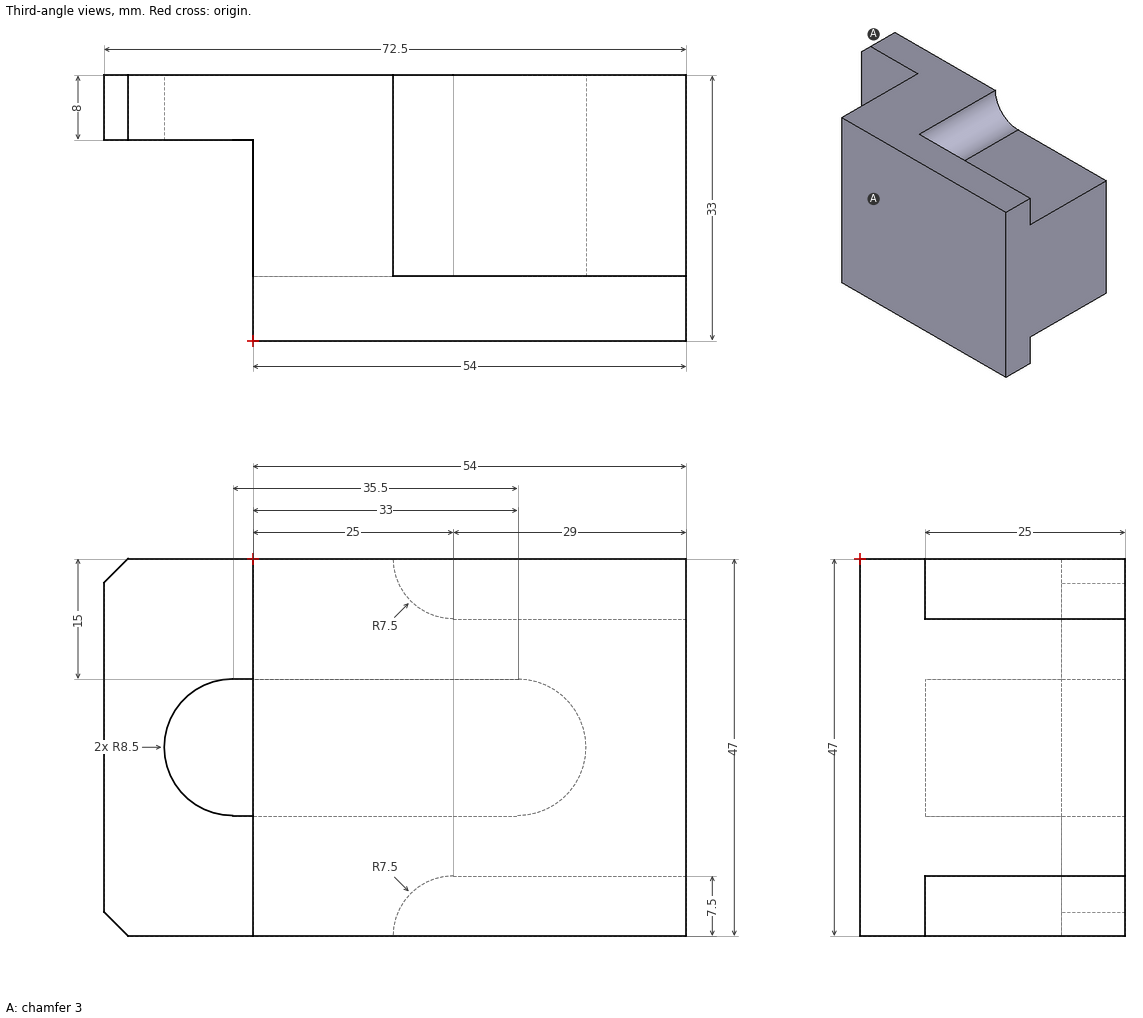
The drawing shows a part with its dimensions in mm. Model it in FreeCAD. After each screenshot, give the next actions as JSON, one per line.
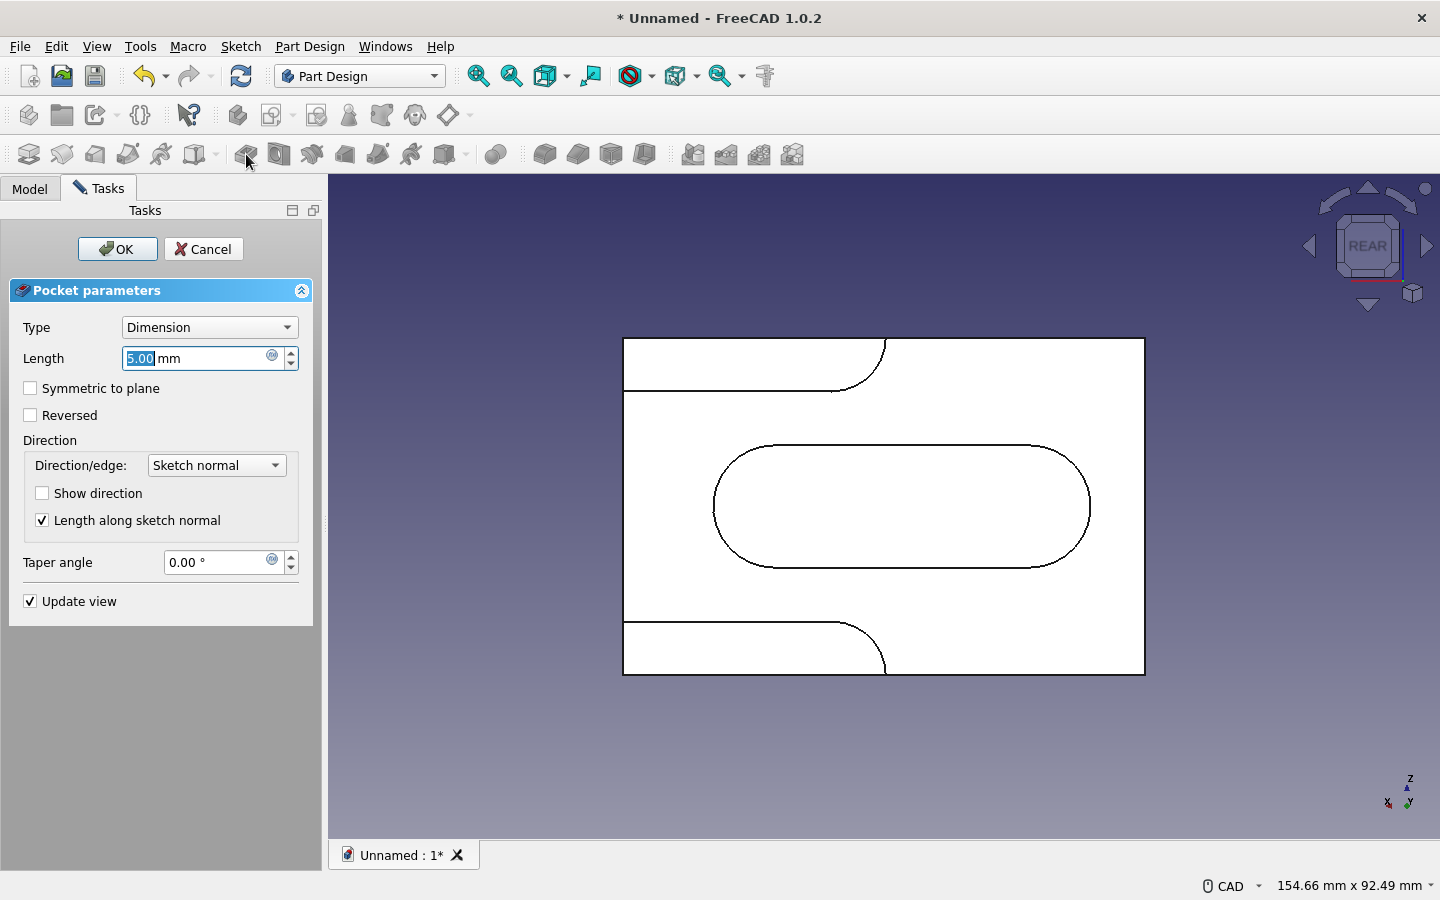
{"action": "type", "text": "25"}
{"action": "key", "text": "Tab"}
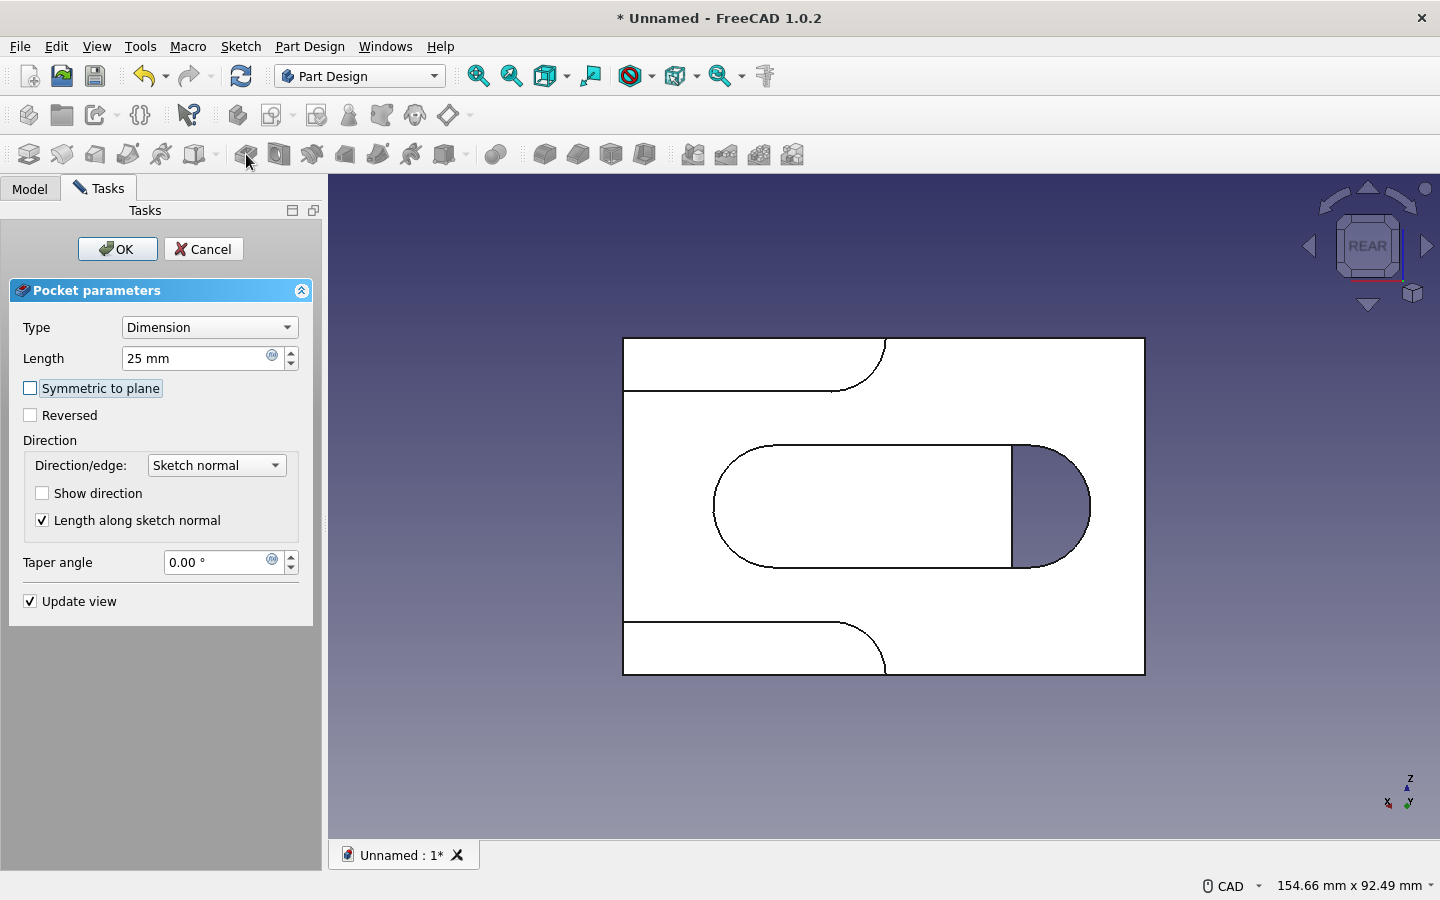
{"action": "left_click", "coordinate": [118, 249]}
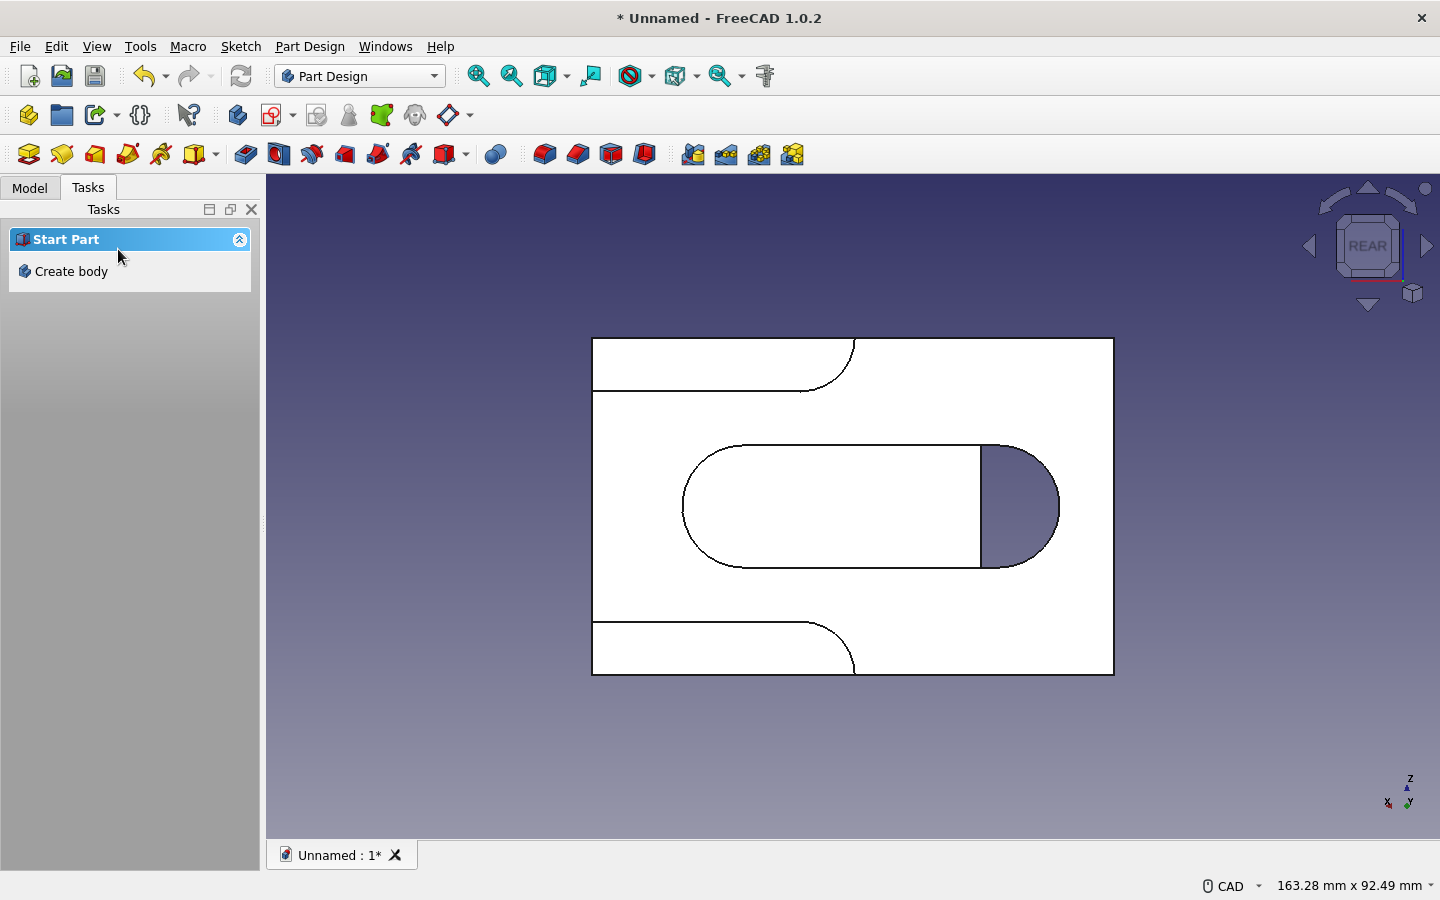
{"action": "key", "text": "0"}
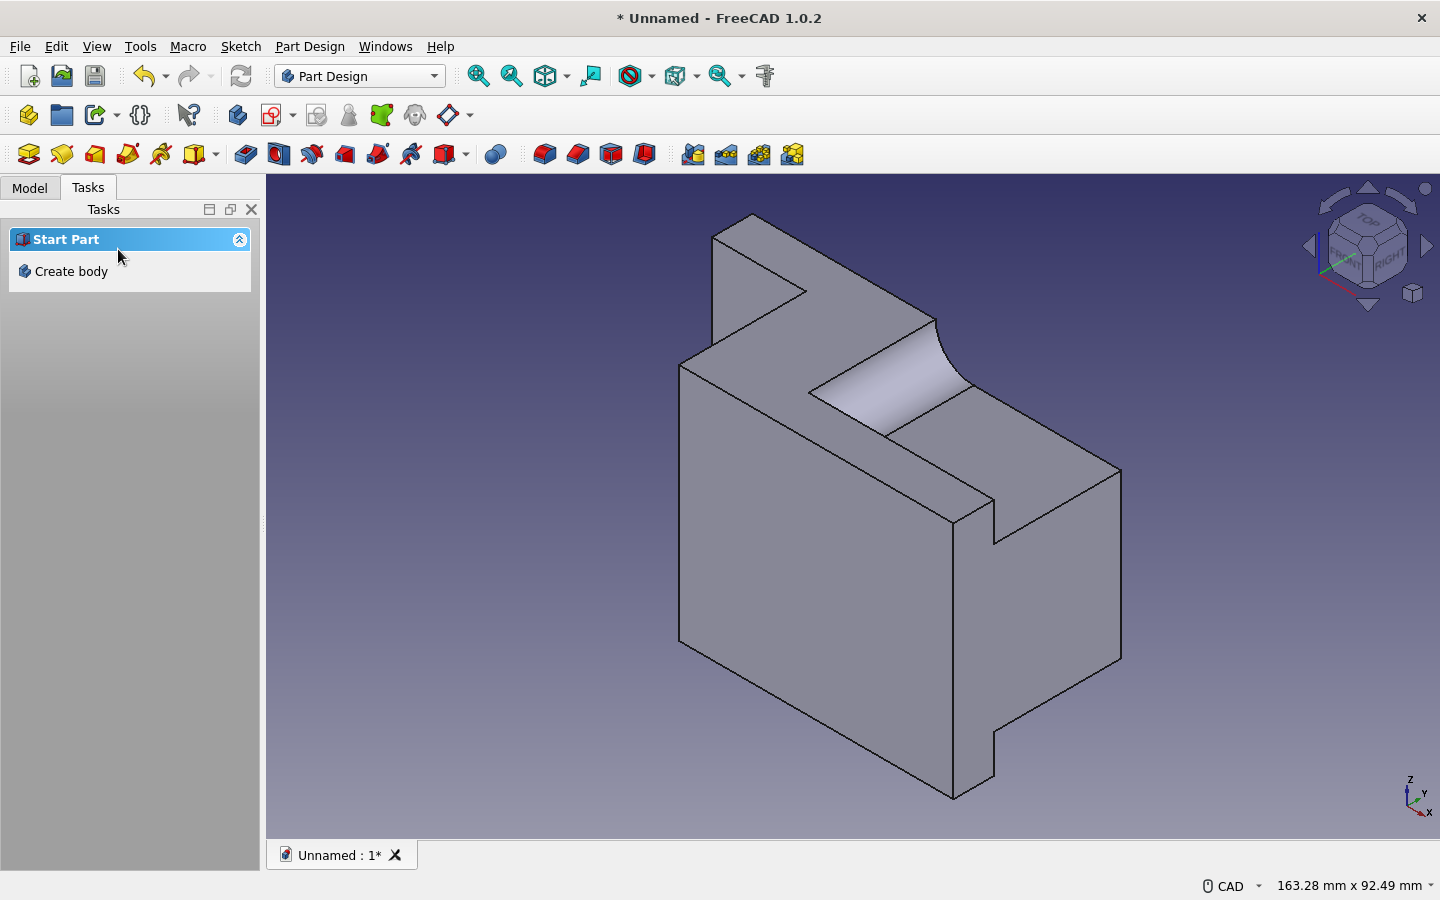
{"action": "key", "text": "2"}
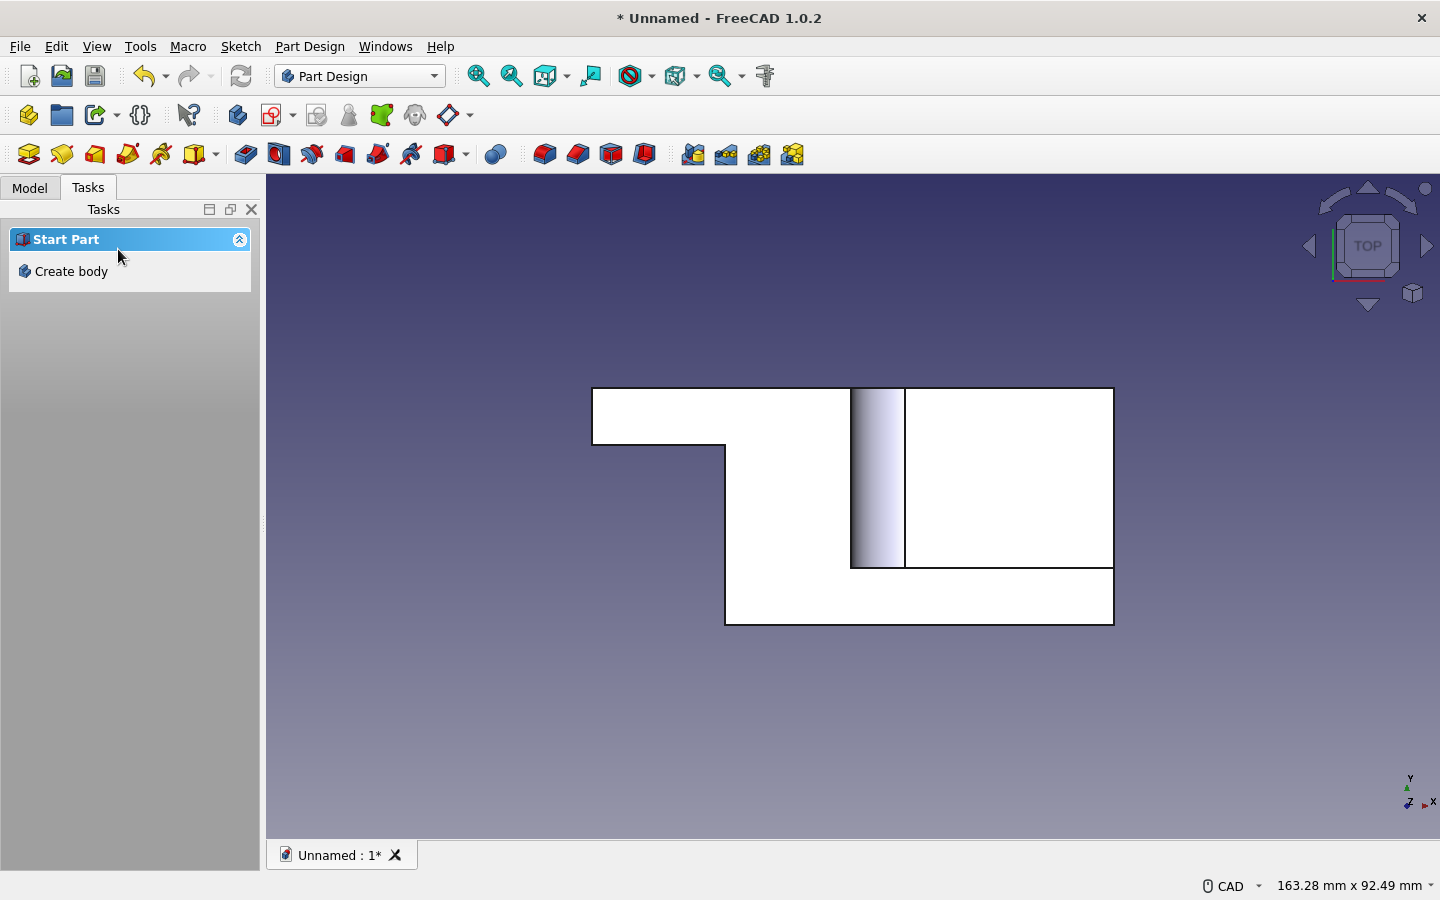
{"action": "key", "text": "v f"}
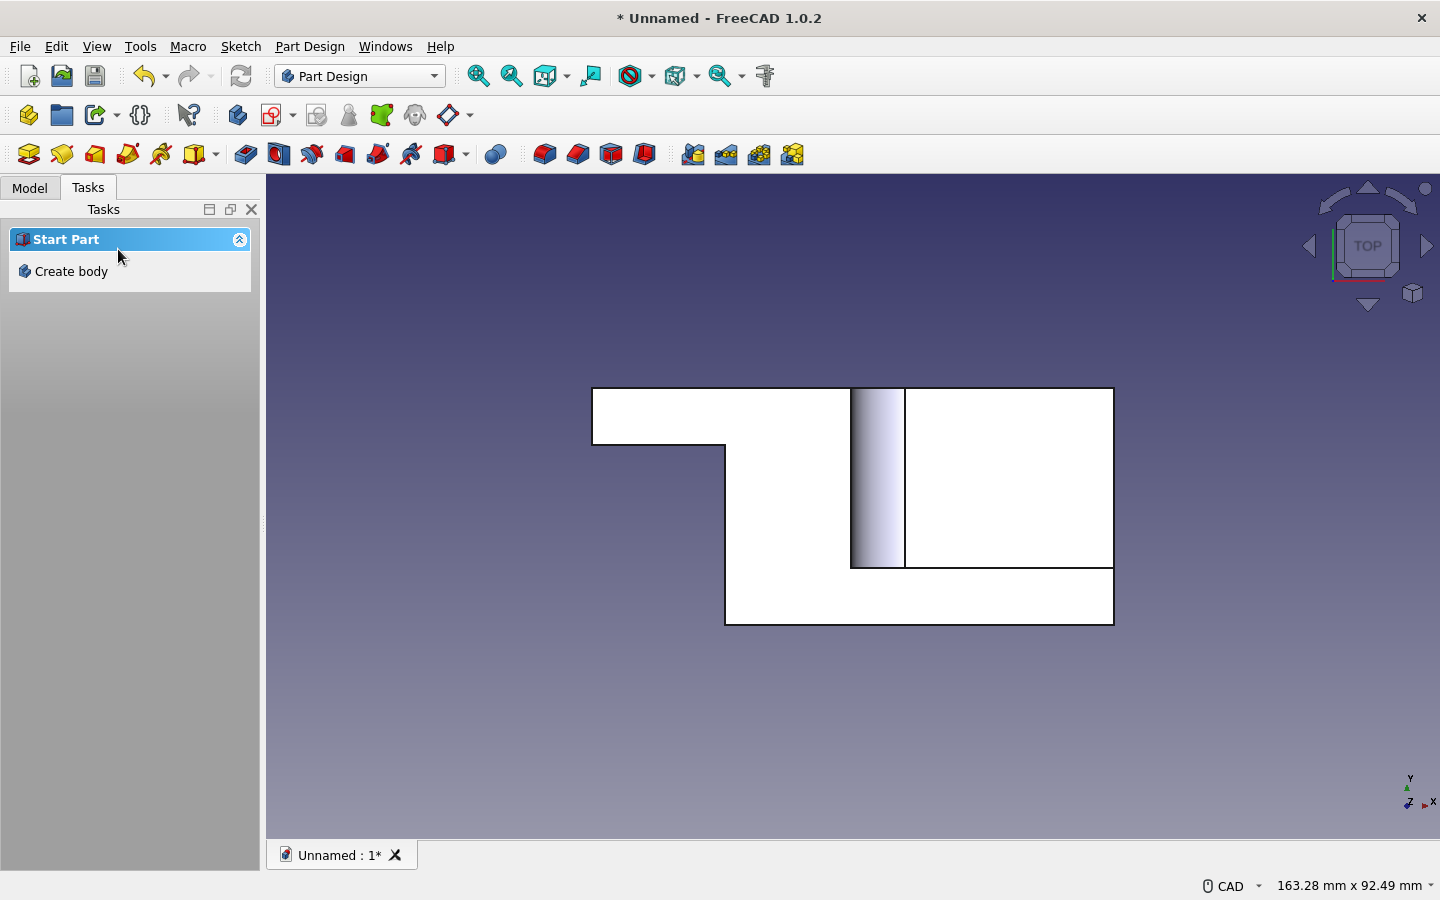
{"action": "left_click", "coordinate": [592, 416]}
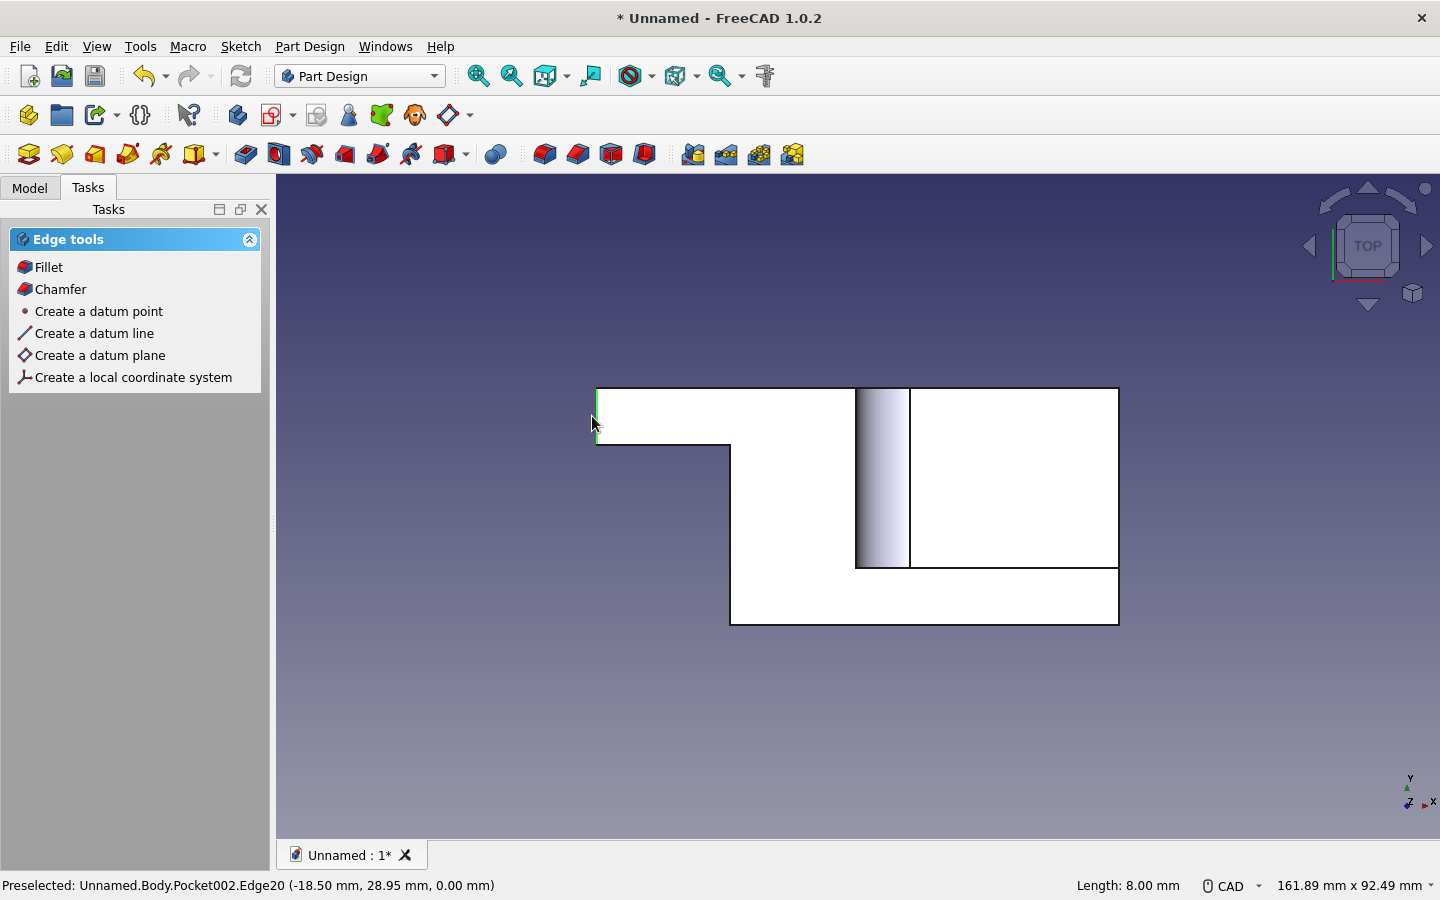
{"action": "key", "text": "1"}